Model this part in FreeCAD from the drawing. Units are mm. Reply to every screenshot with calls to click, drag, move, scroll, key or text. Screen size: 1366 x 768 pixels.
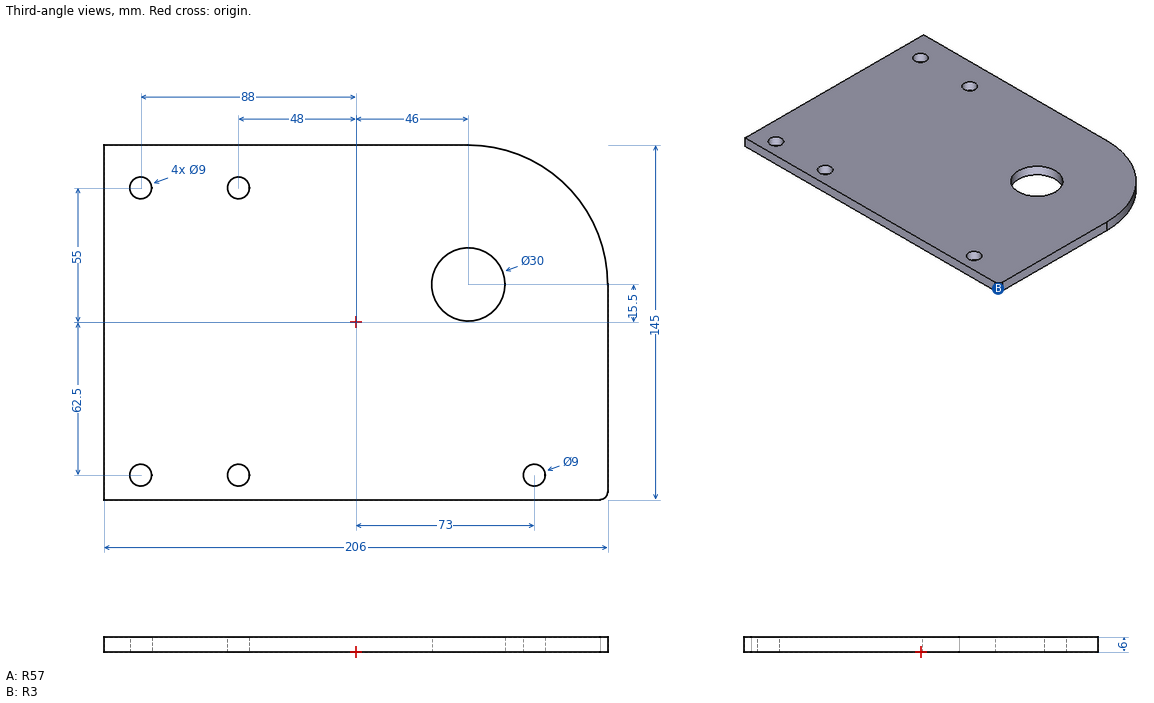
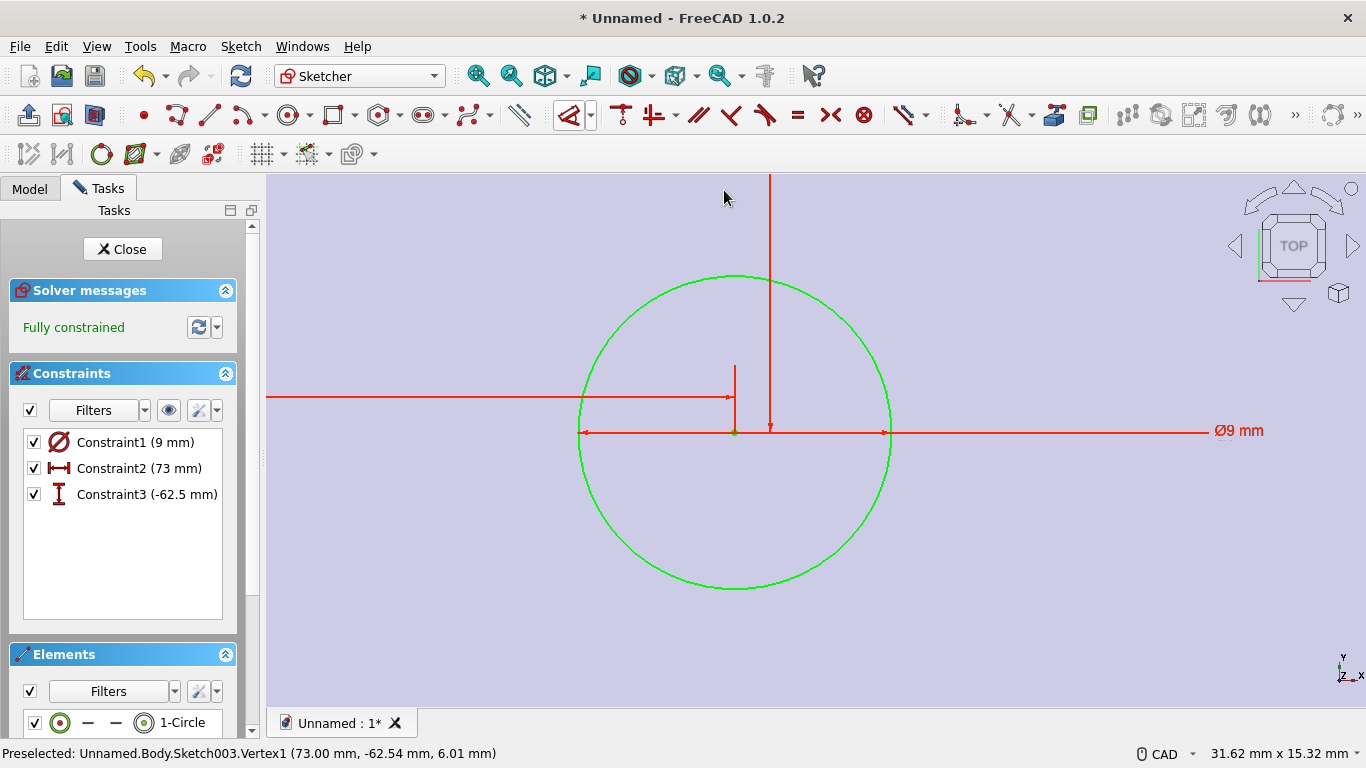
click(123, 249)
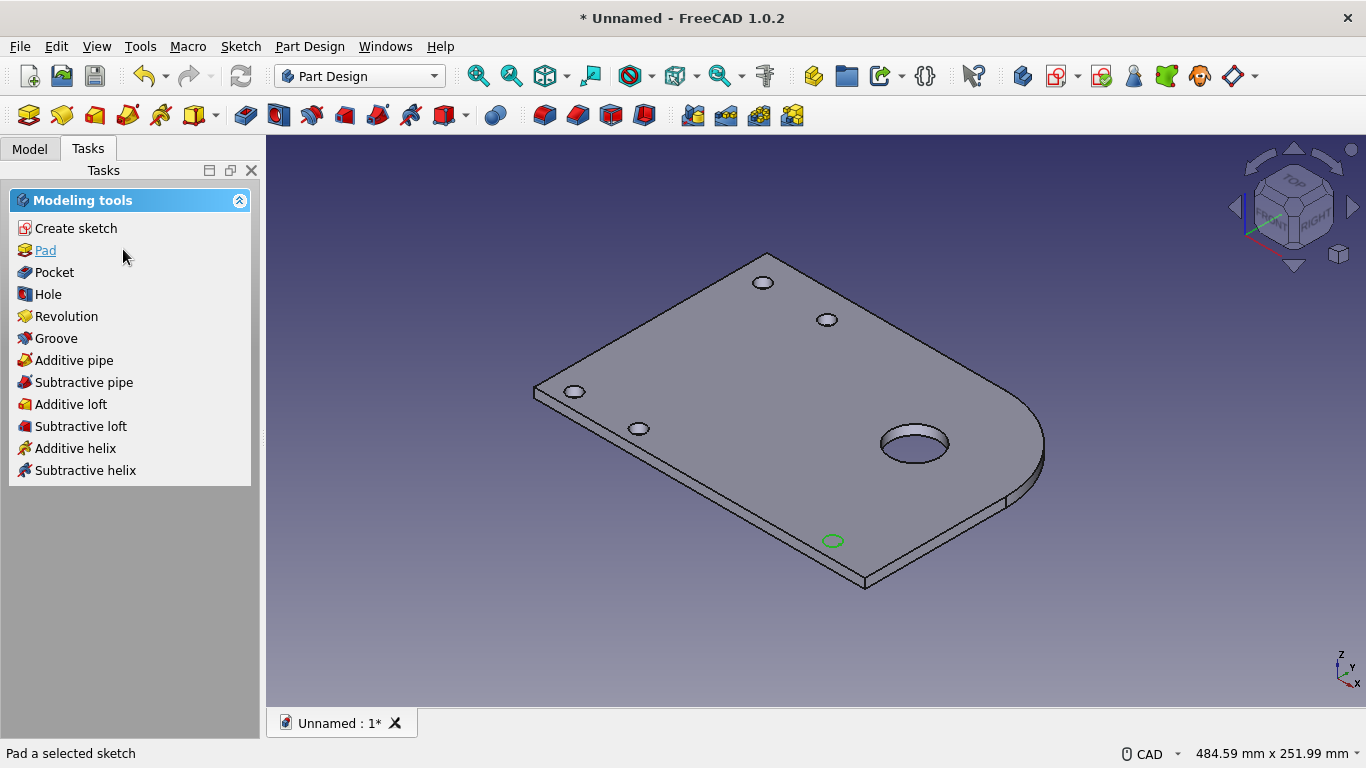
click(246, 116)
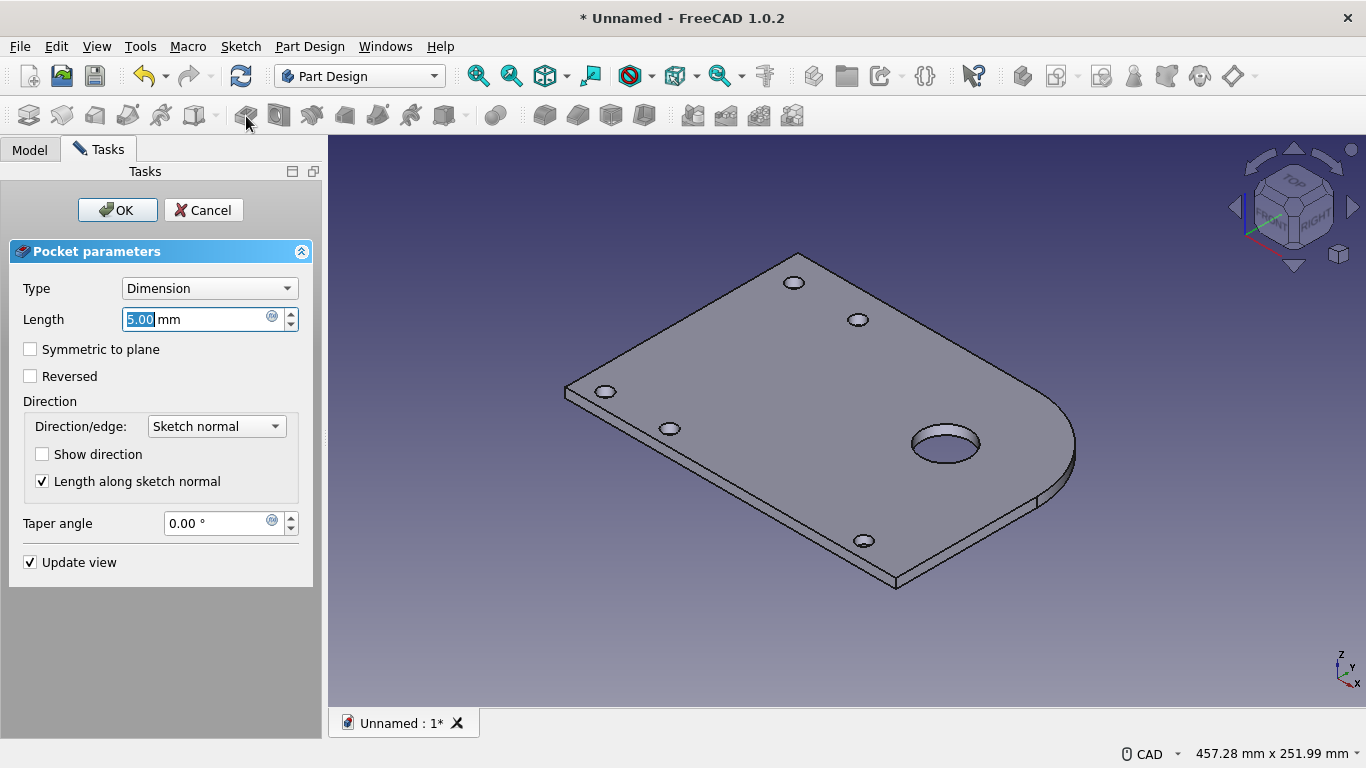
click(210, 288)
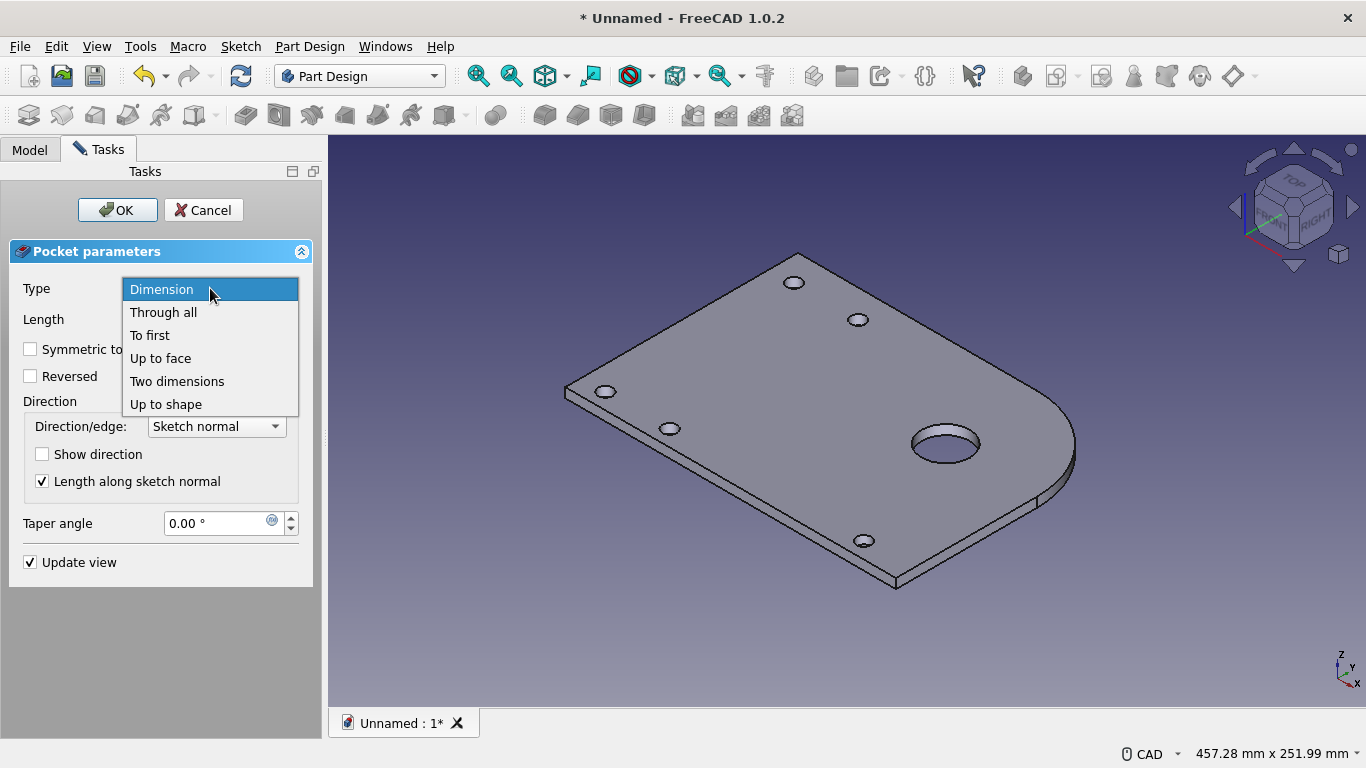
click(208, 312)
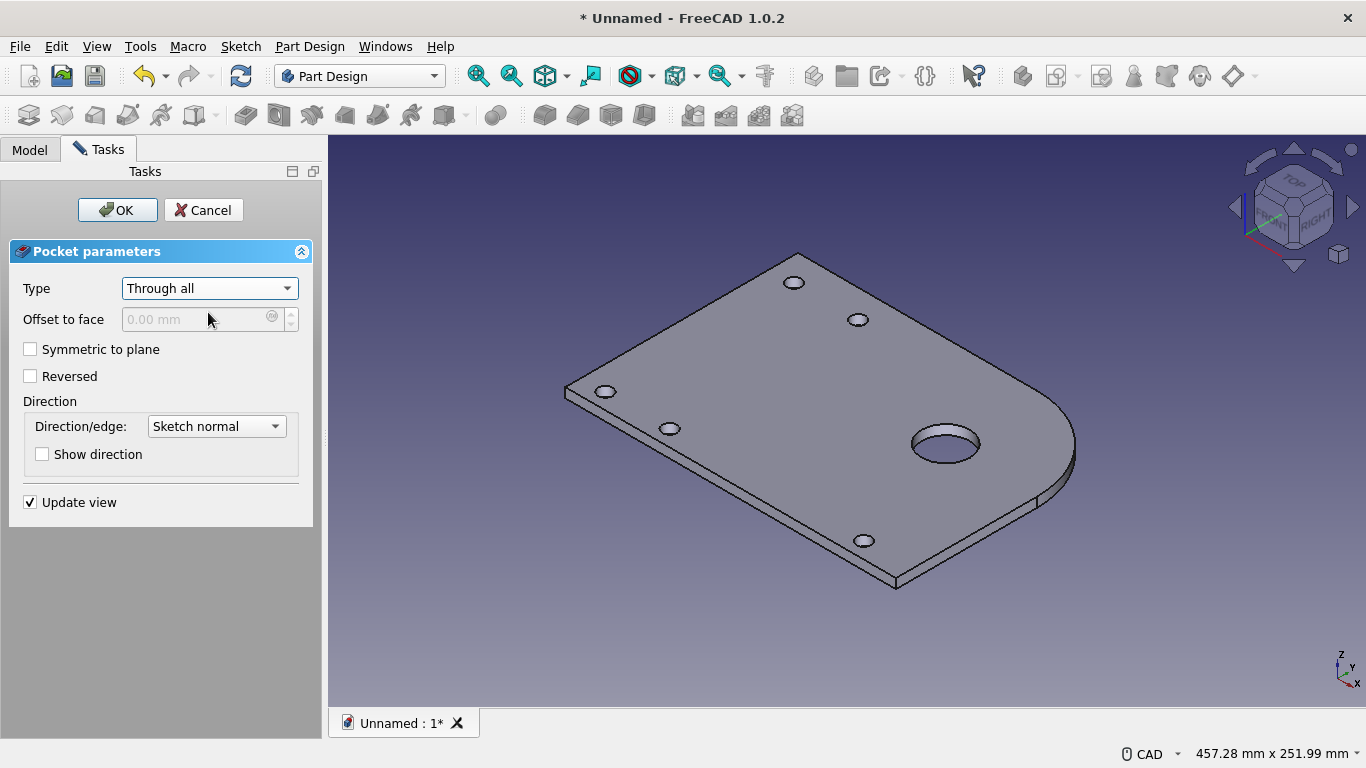
click(118, 210)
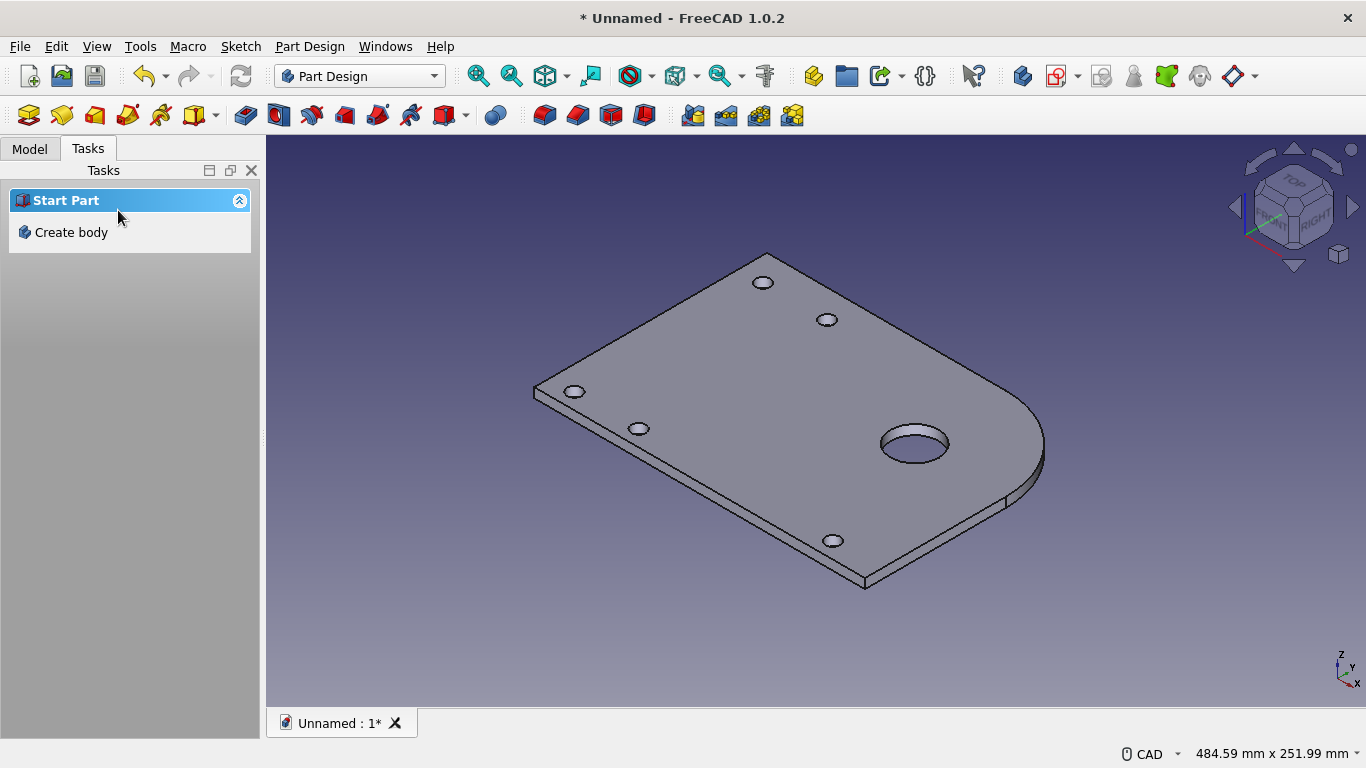
click(865, 583)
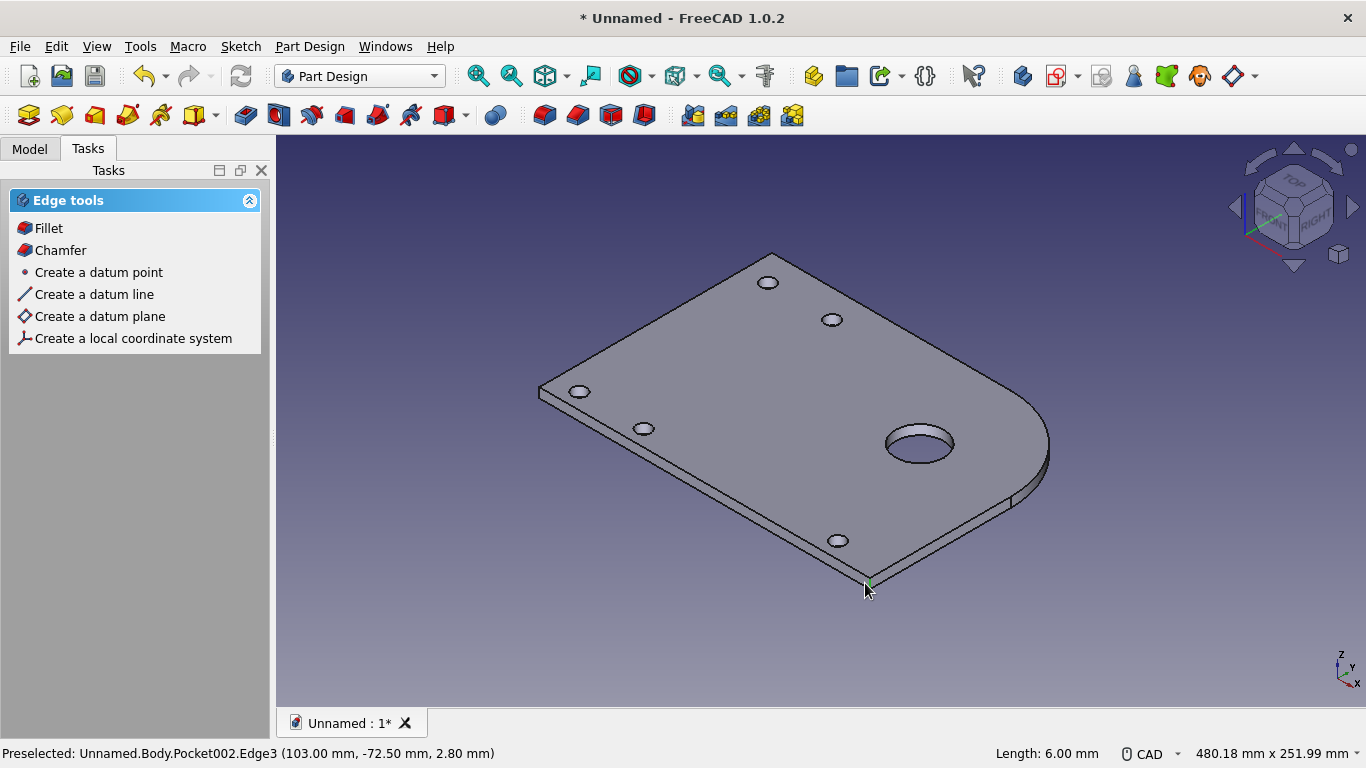
click(545, 116)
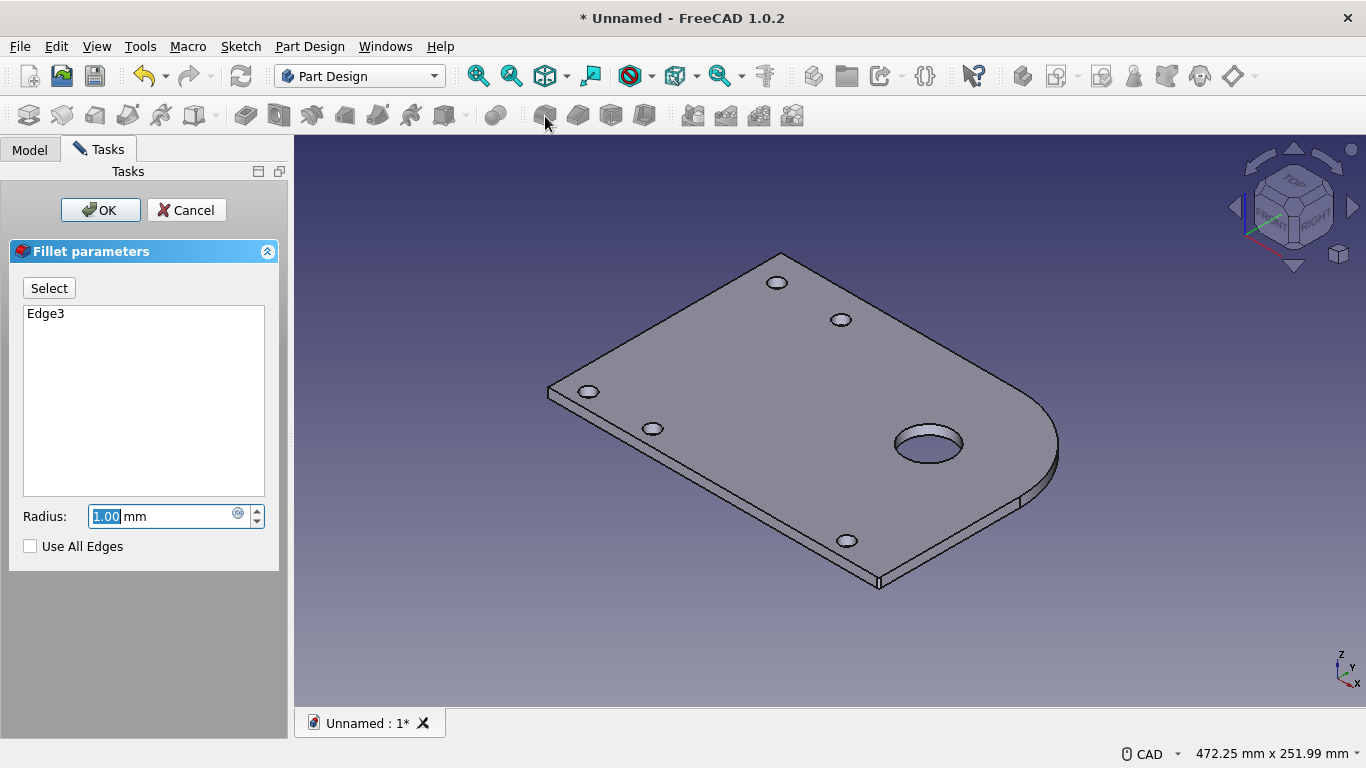
text(3)
key(Tab)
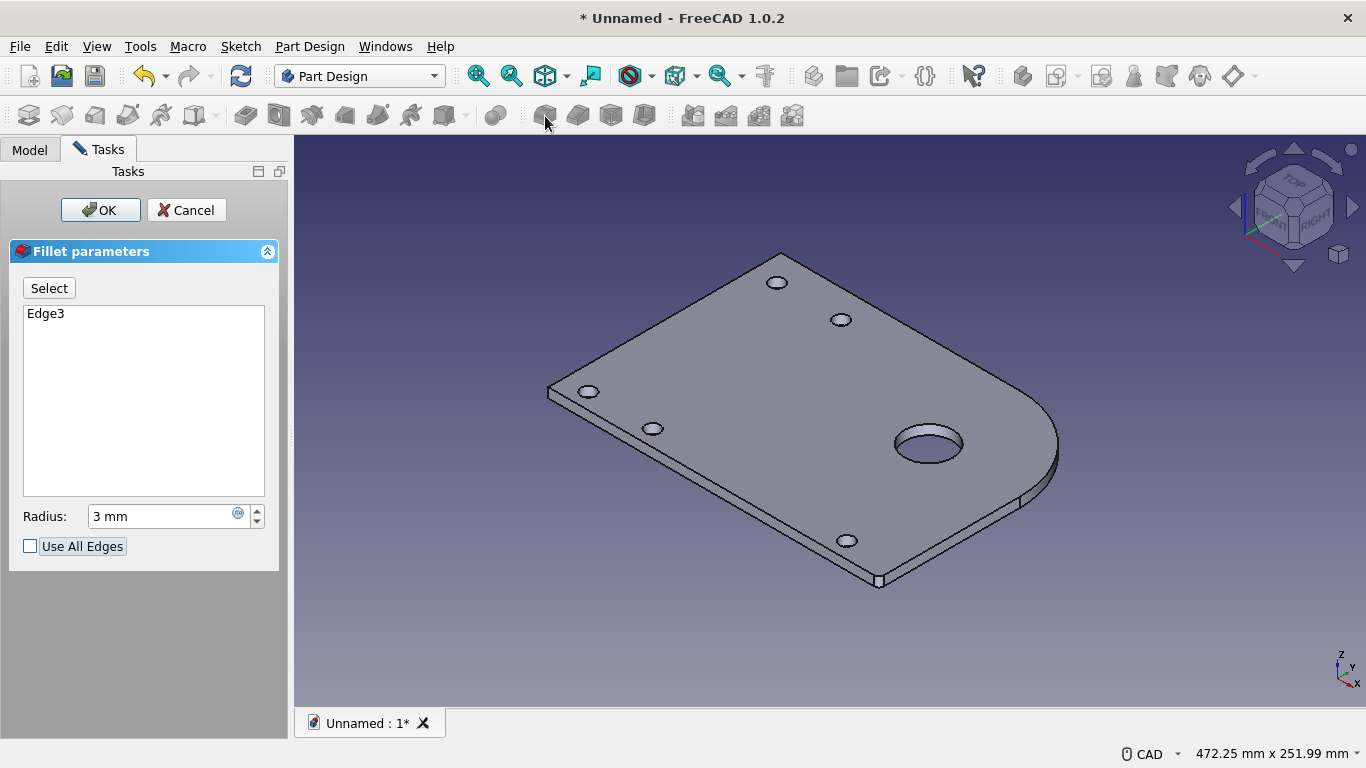
click(101, 210)